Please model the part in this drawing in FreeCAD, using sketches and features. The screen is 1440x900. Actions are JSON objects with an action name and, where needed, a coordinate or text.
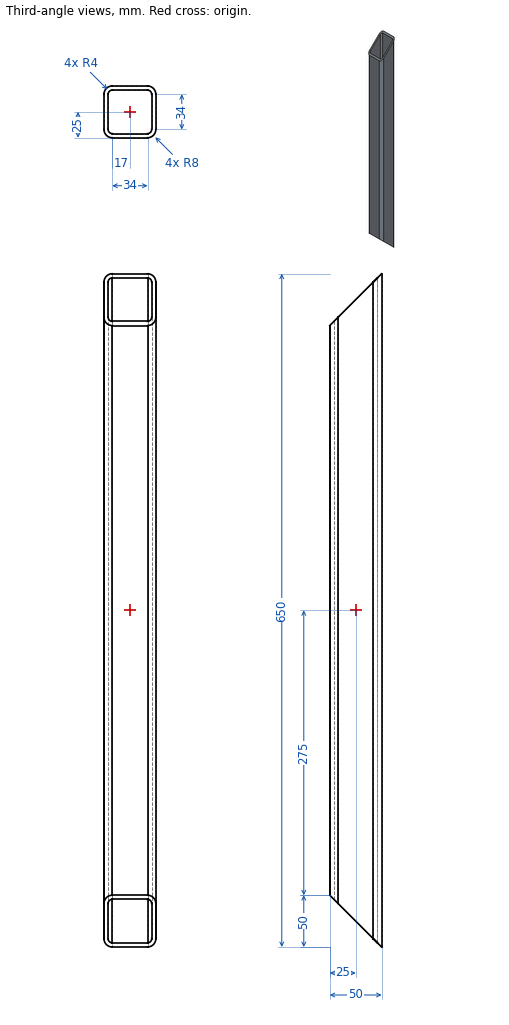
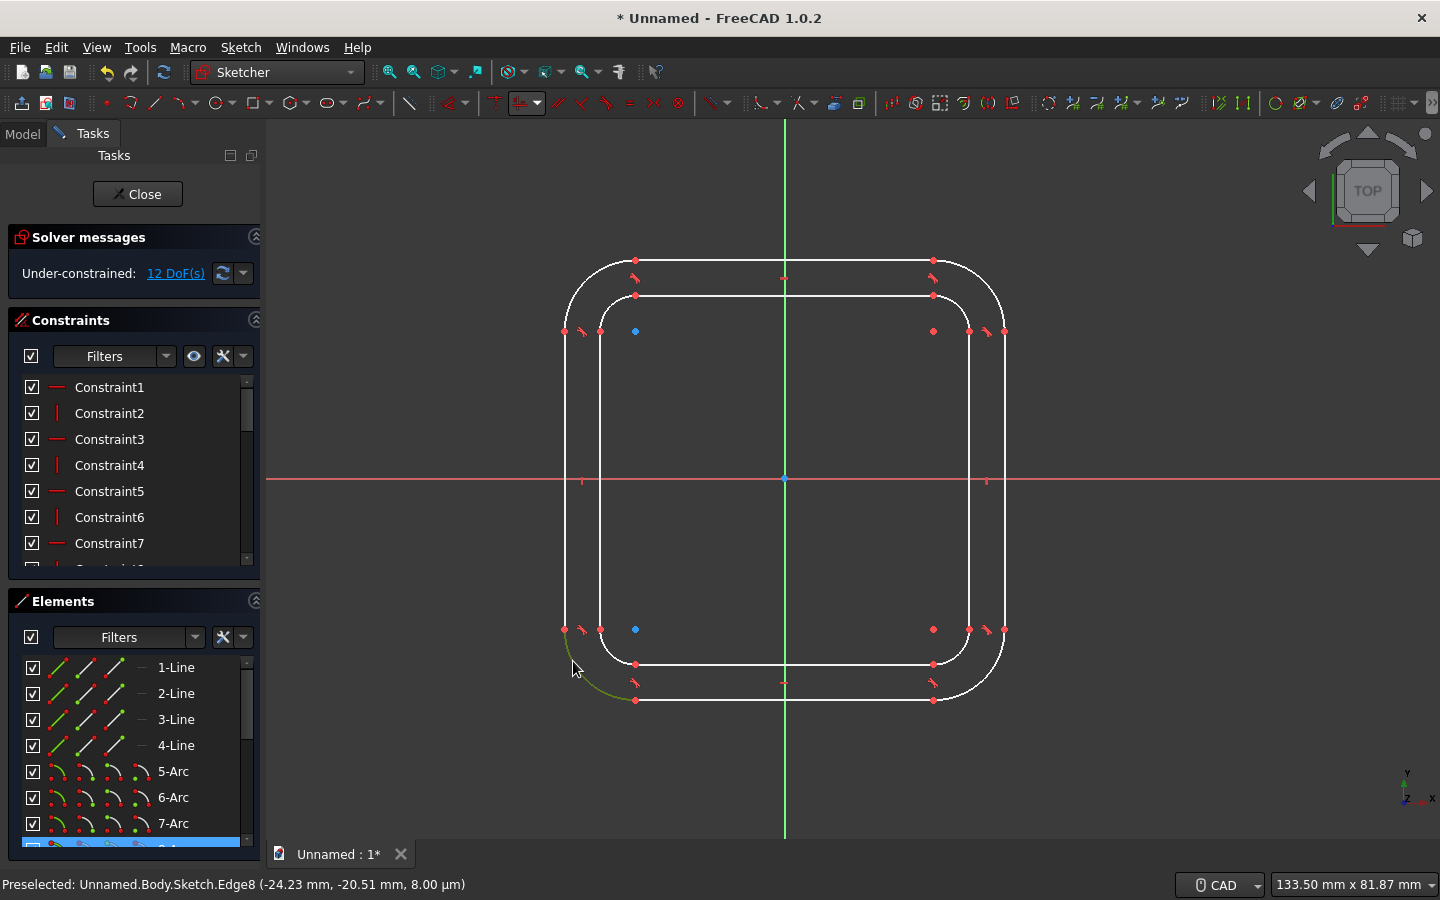
{"action": "left_click", "coordinate": [604, 645]}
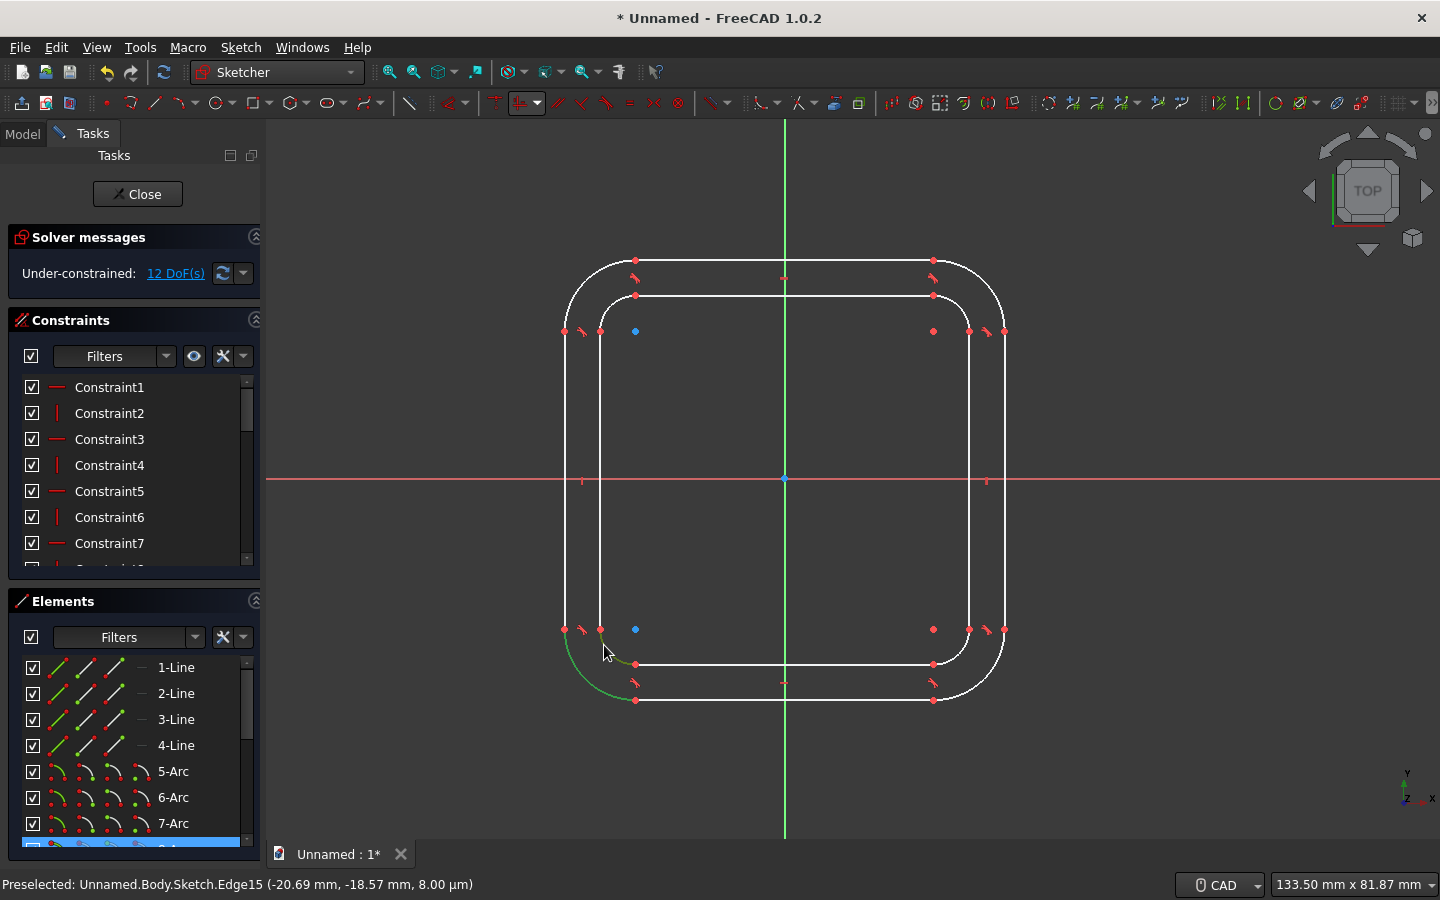
{"action": "key", "text": "c"}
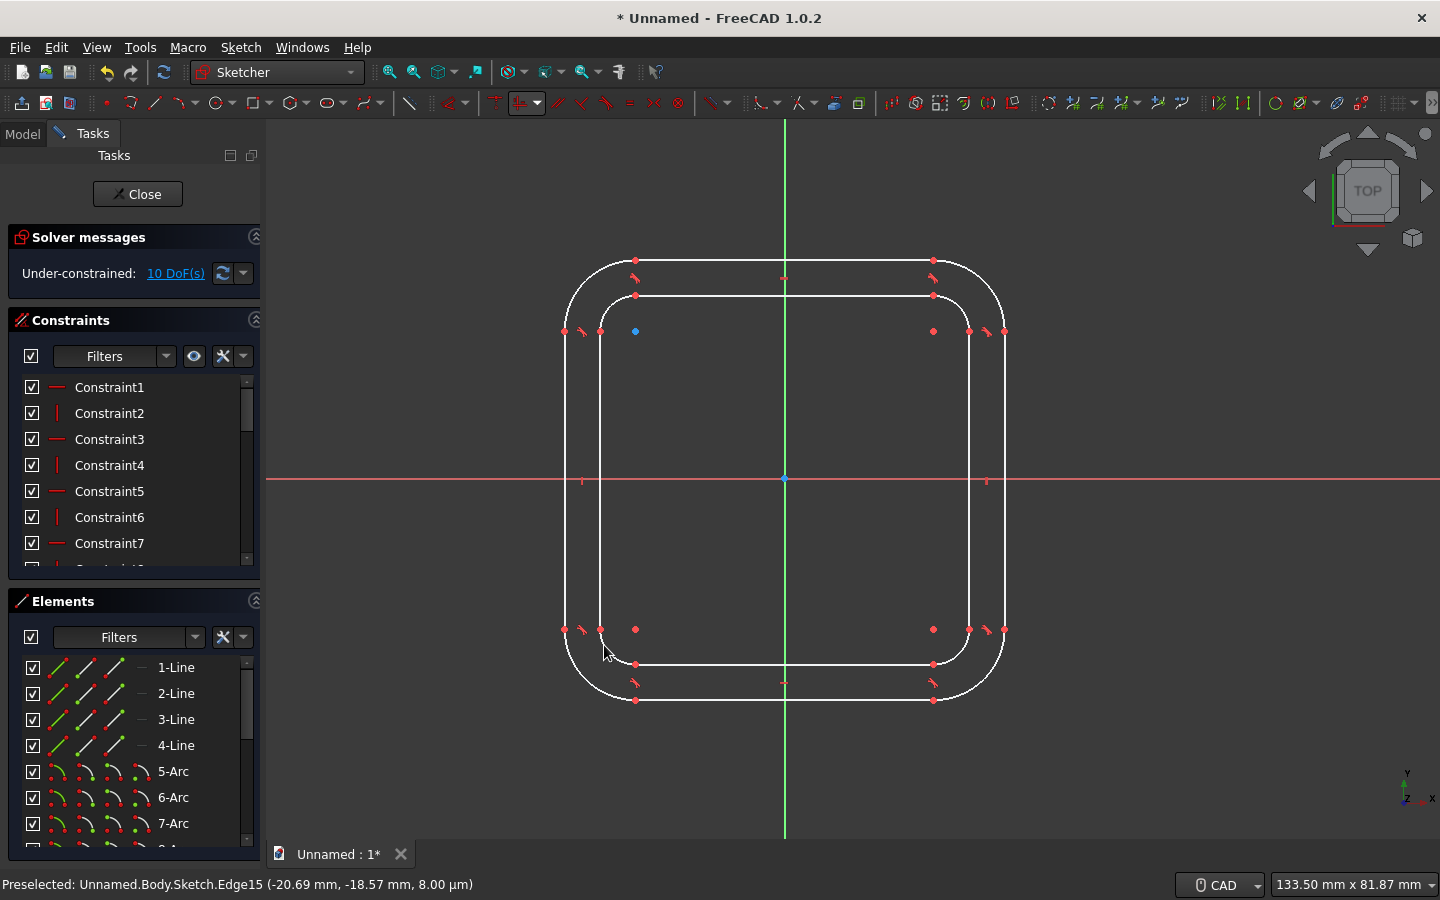
{"action": "left_click", "coordinate": [966, 692]}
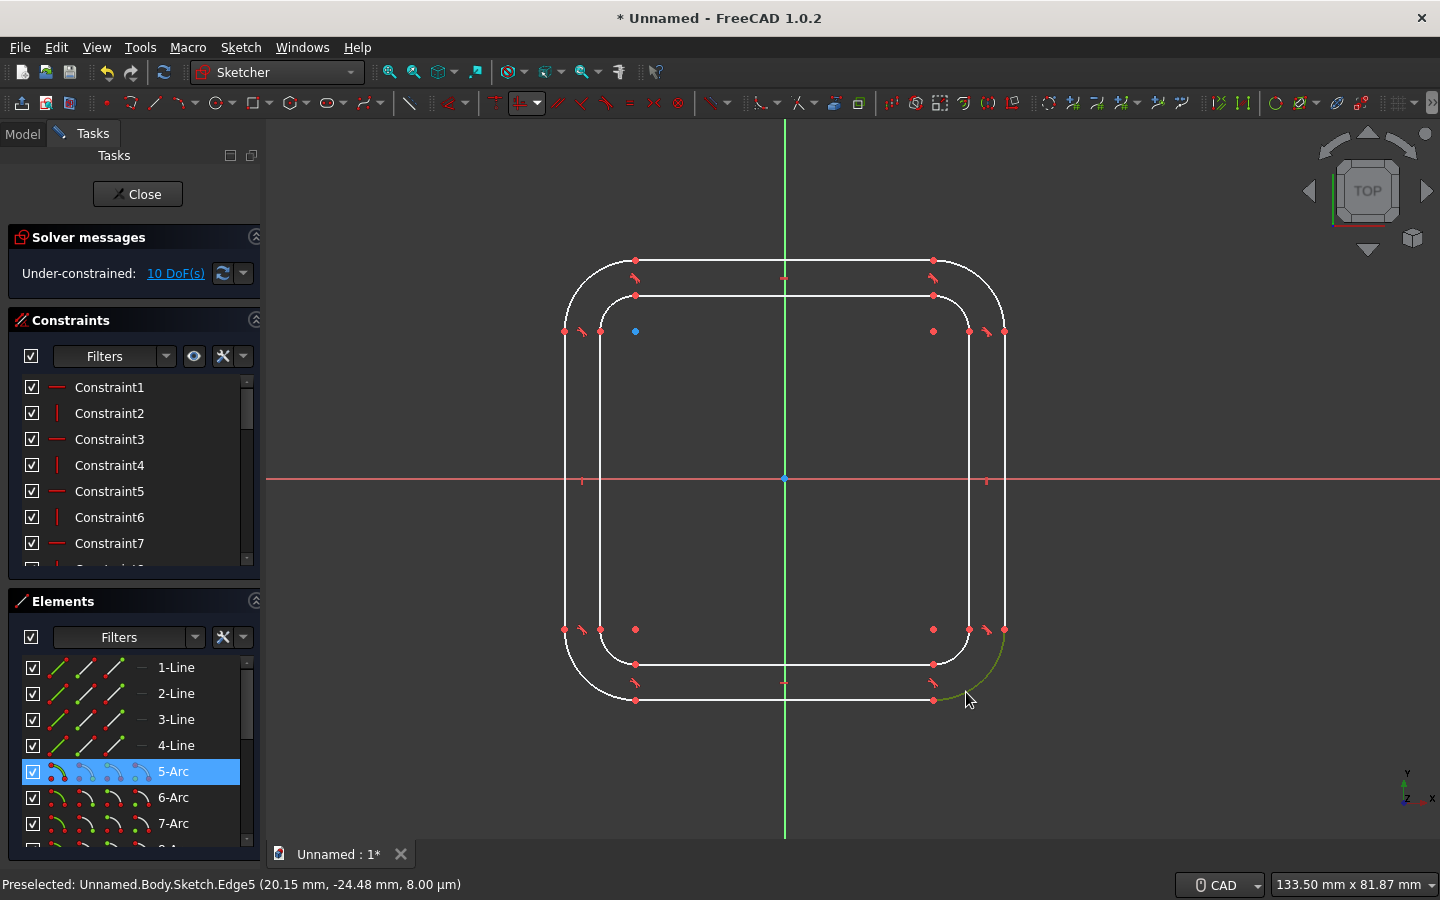
{"action": "left_click", "coordinate": [997, 299]}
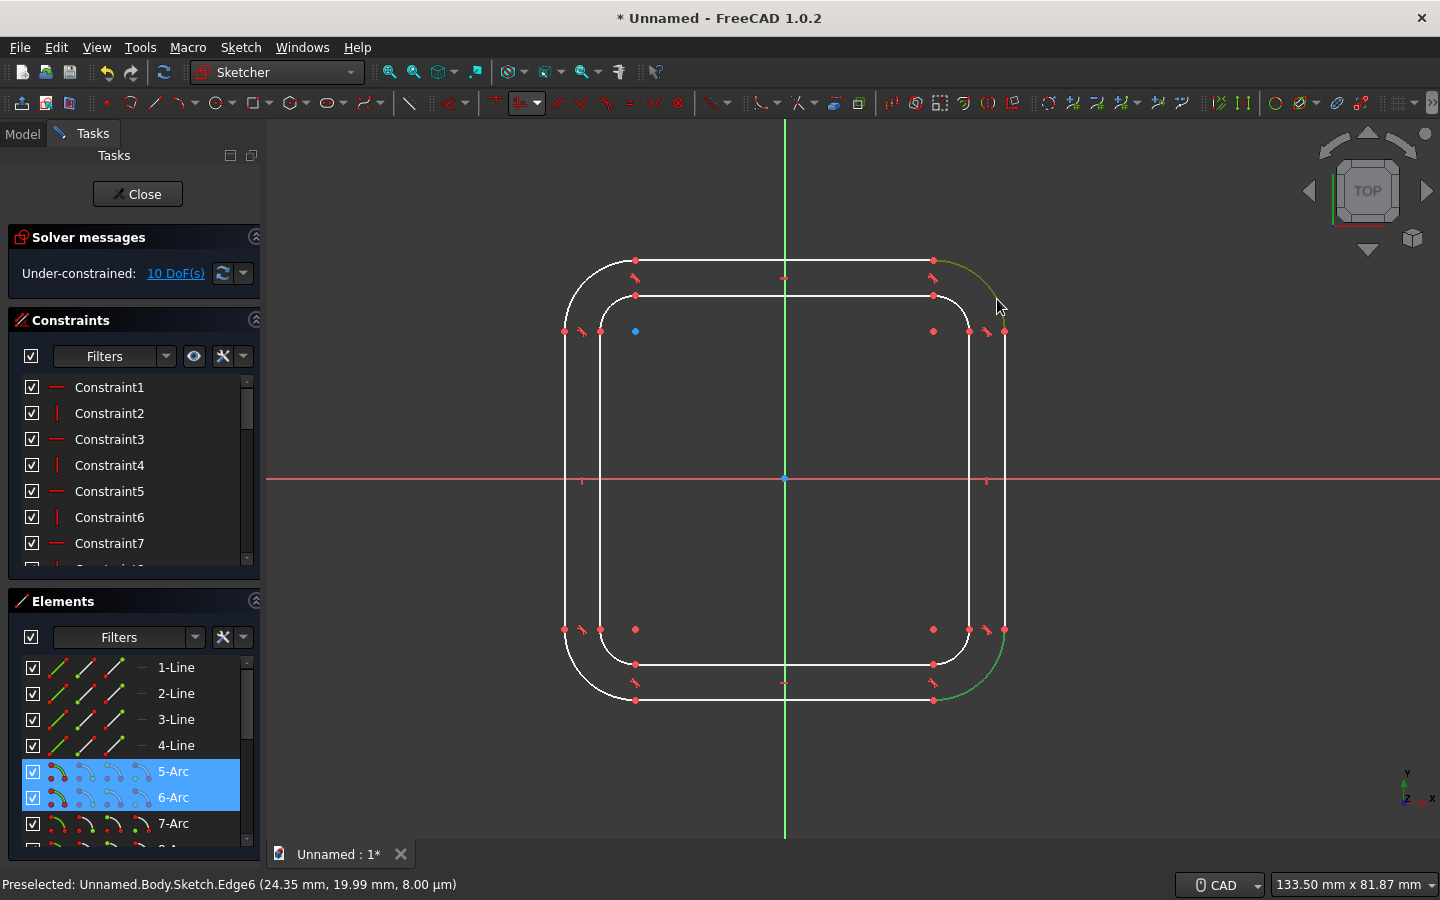
{"action": "left_click", "coordinate": [603, 268]}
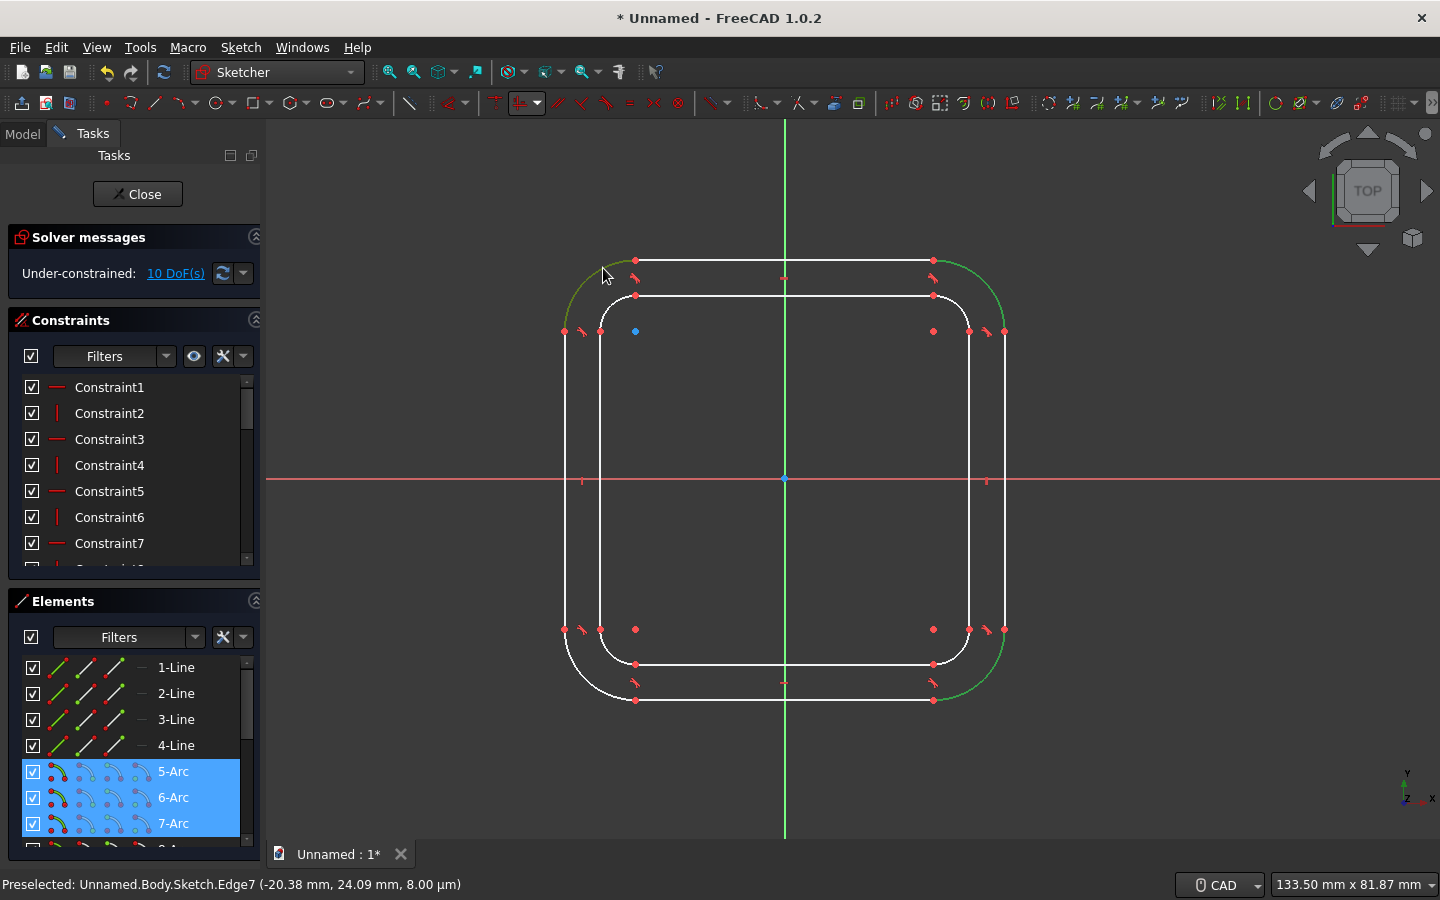
{"action": "left_click", "coordinate": [572, 661]}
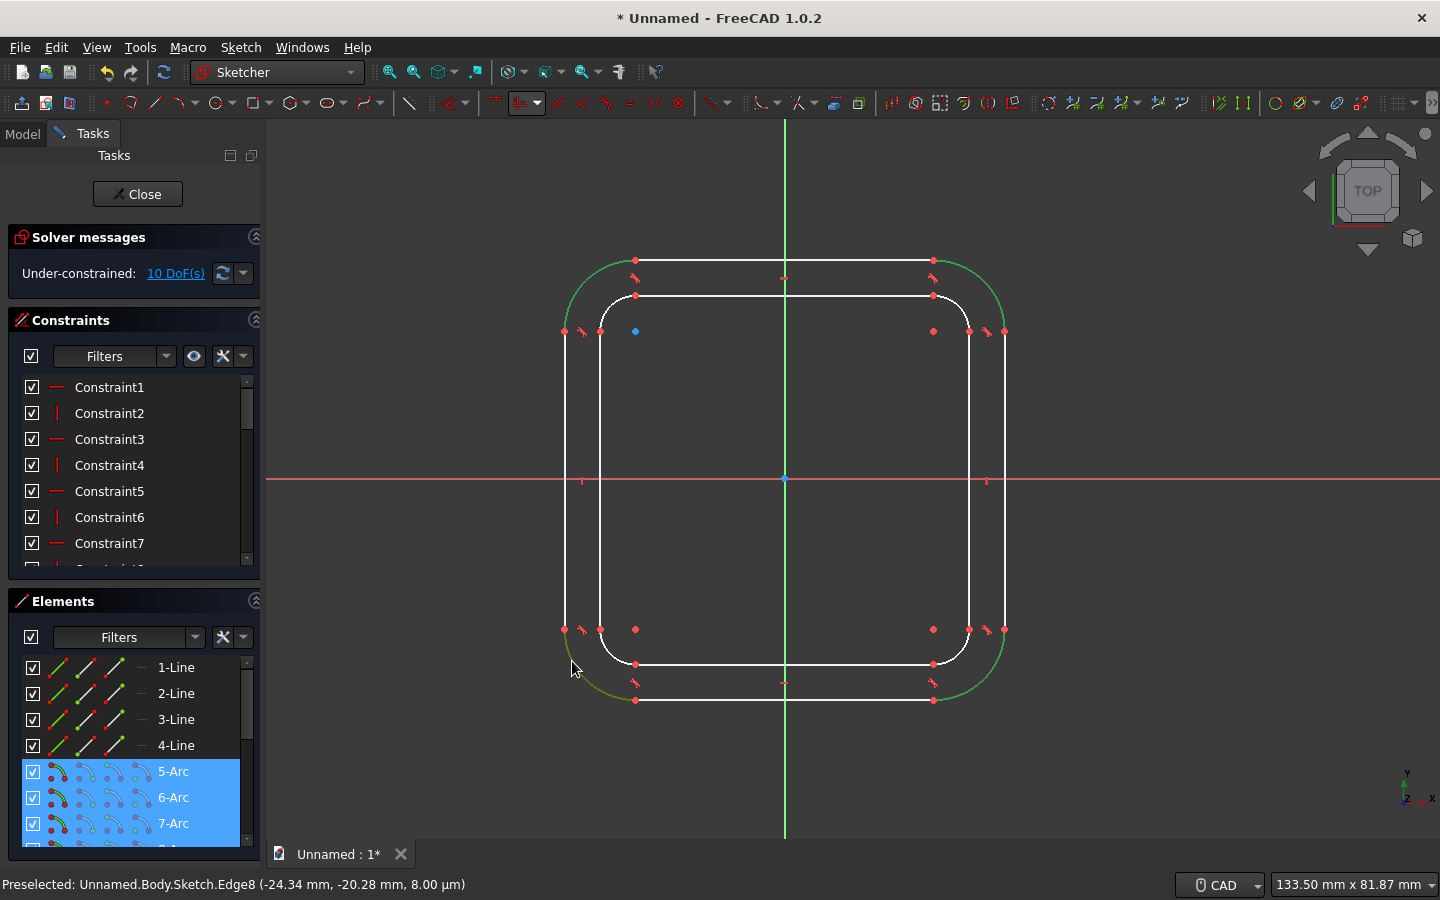
{"action": "key", "text": "e"}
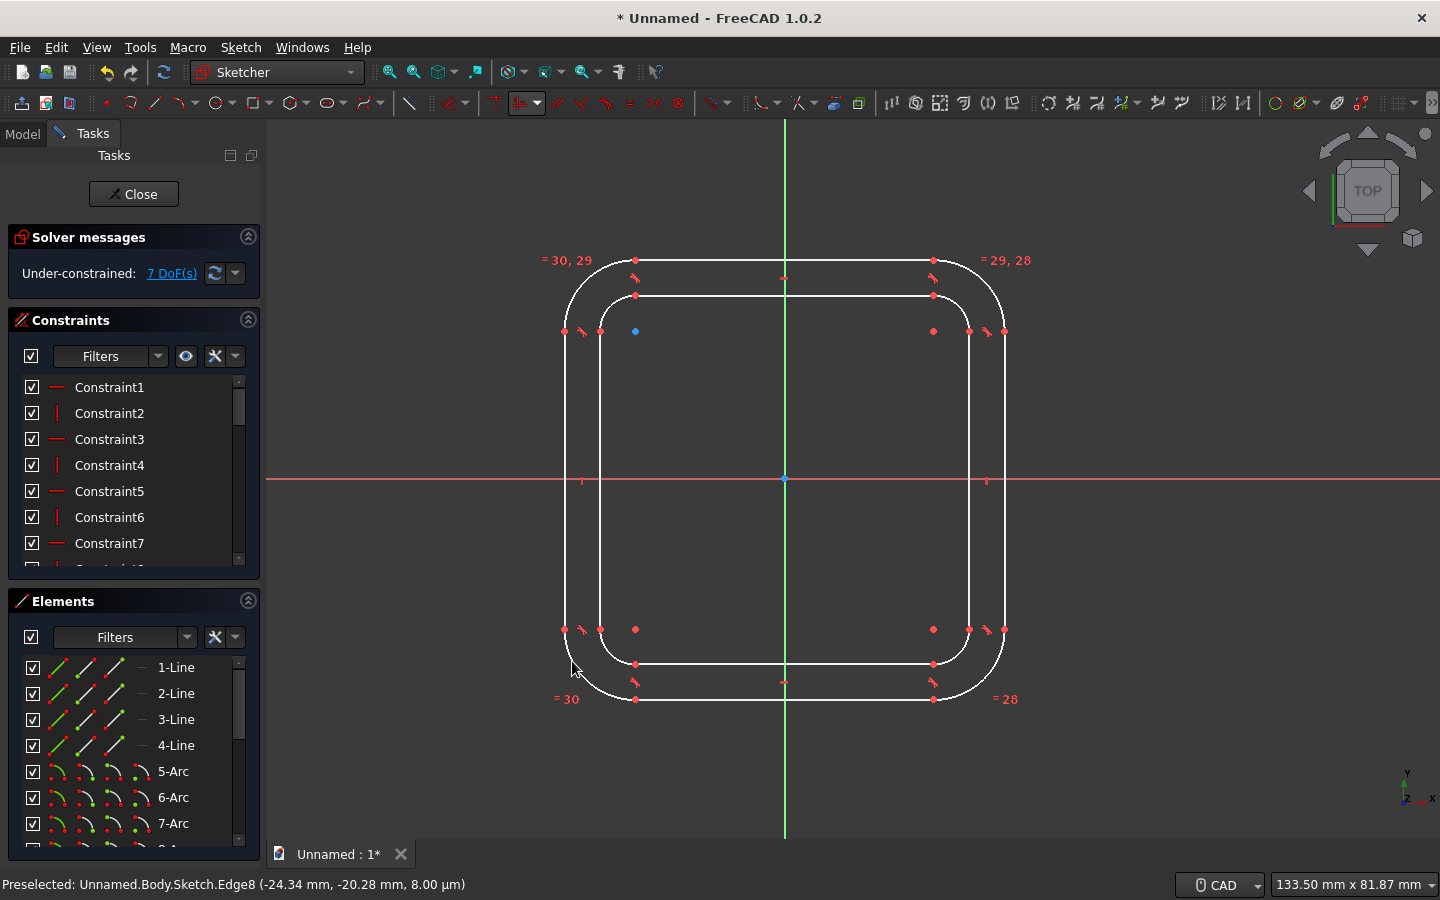
{"action": "left_click", "coordinate": [965, 315]}